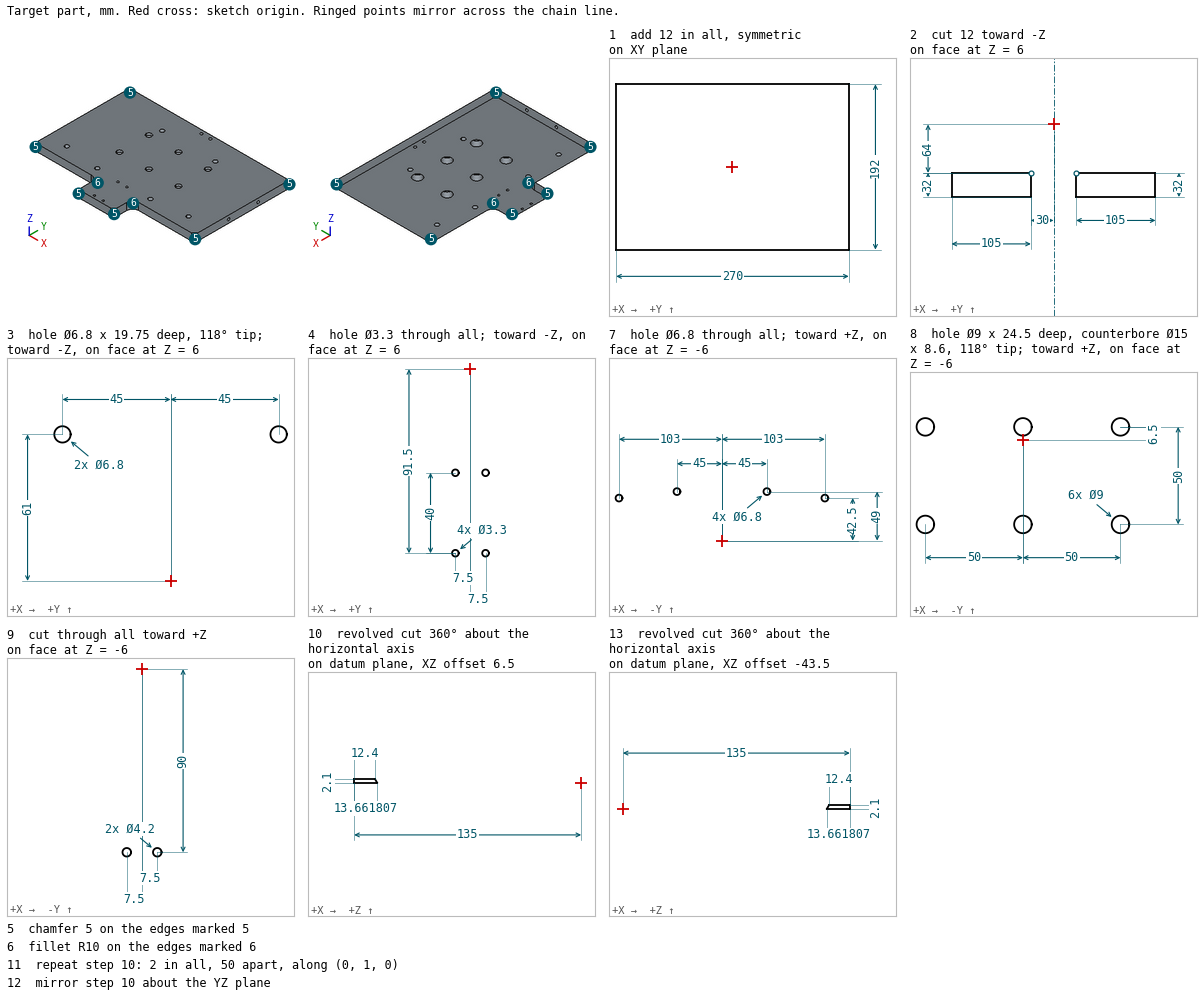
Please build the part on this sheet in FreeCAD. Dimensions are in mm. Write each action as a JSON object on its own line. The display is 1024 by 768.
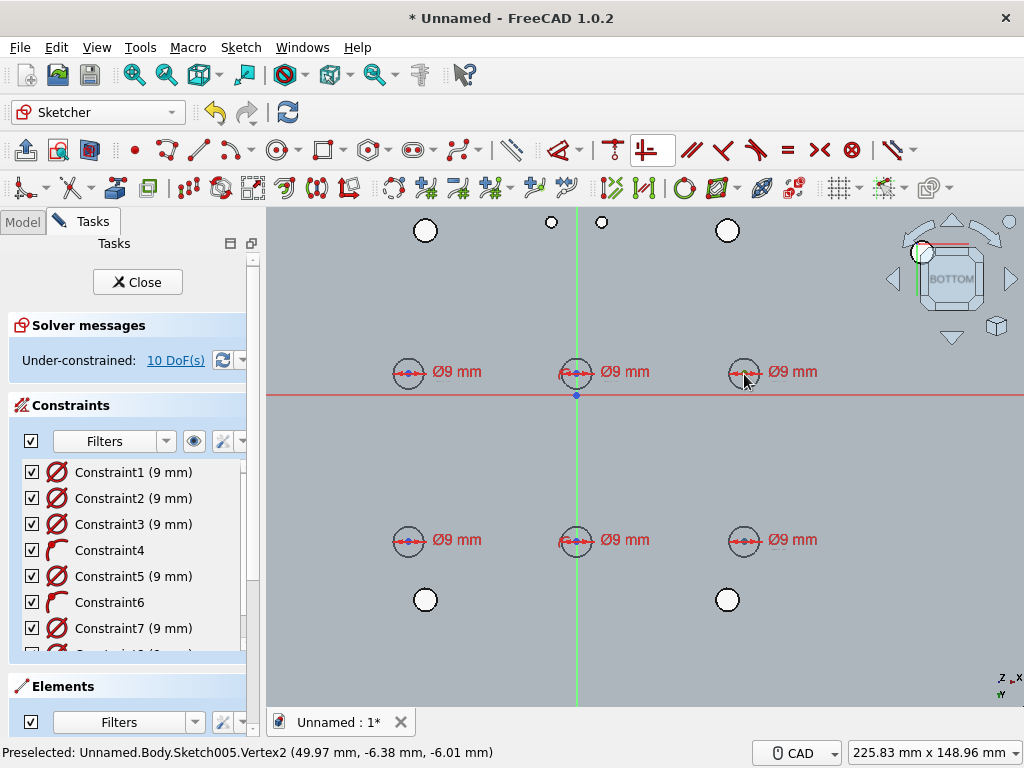
{"action": "key", "text": "v"}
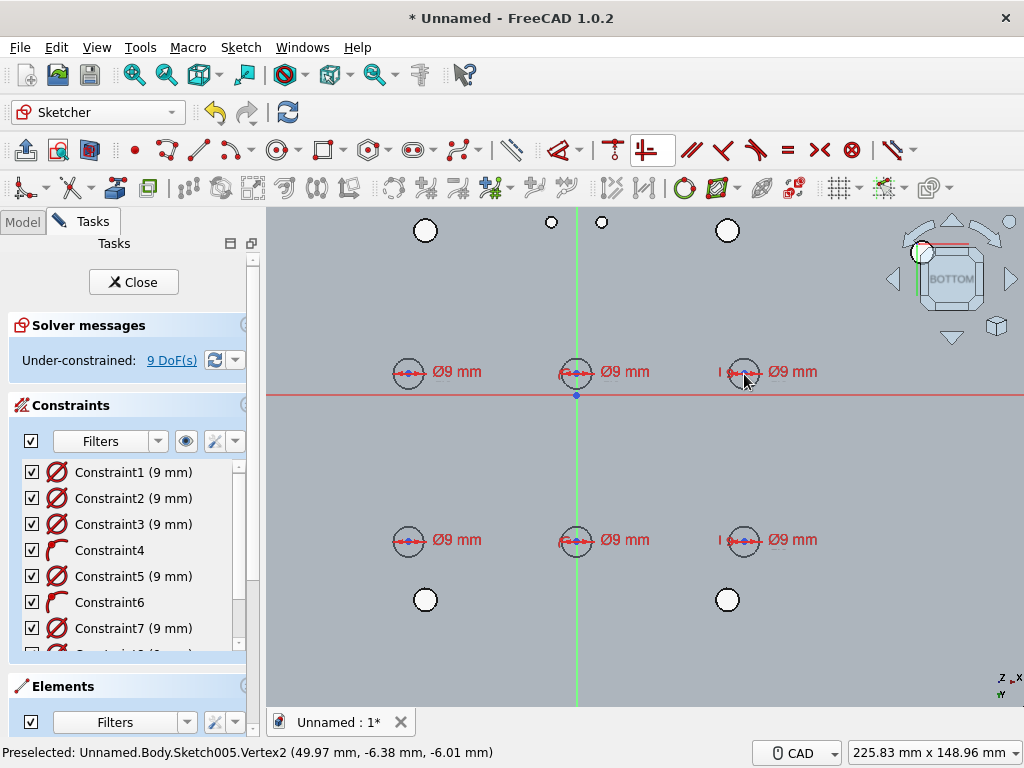
{"action": "left_click", "coordinate": [744, 542]}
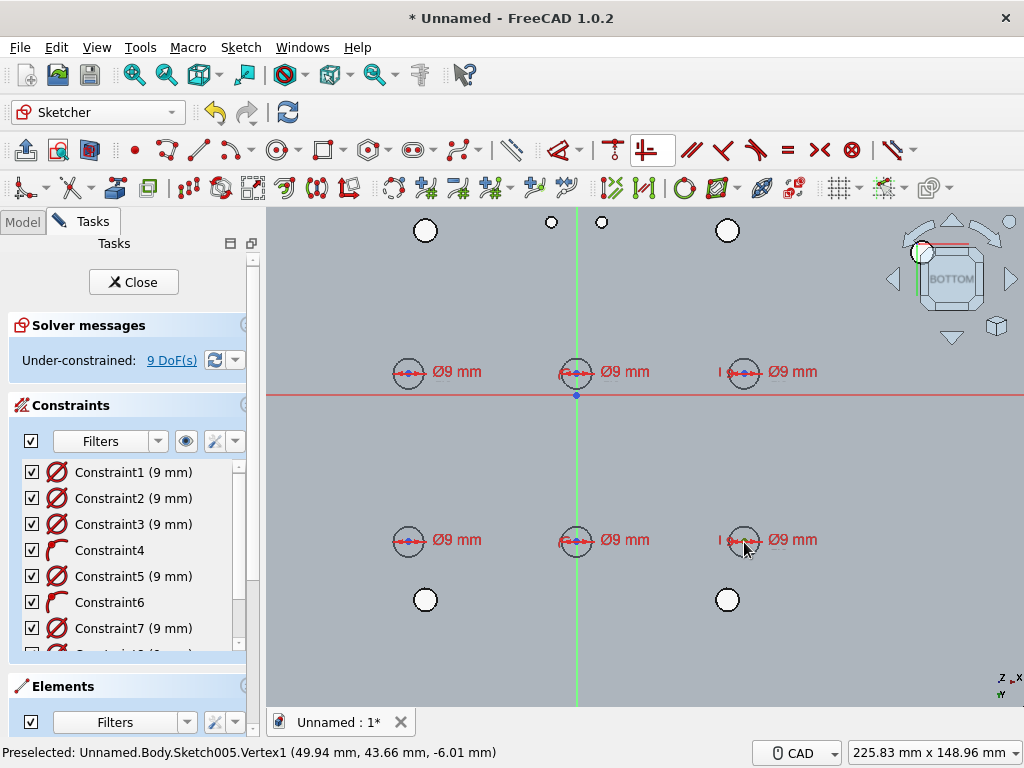
{"action": "left_click", "coordinate": [577, 542]}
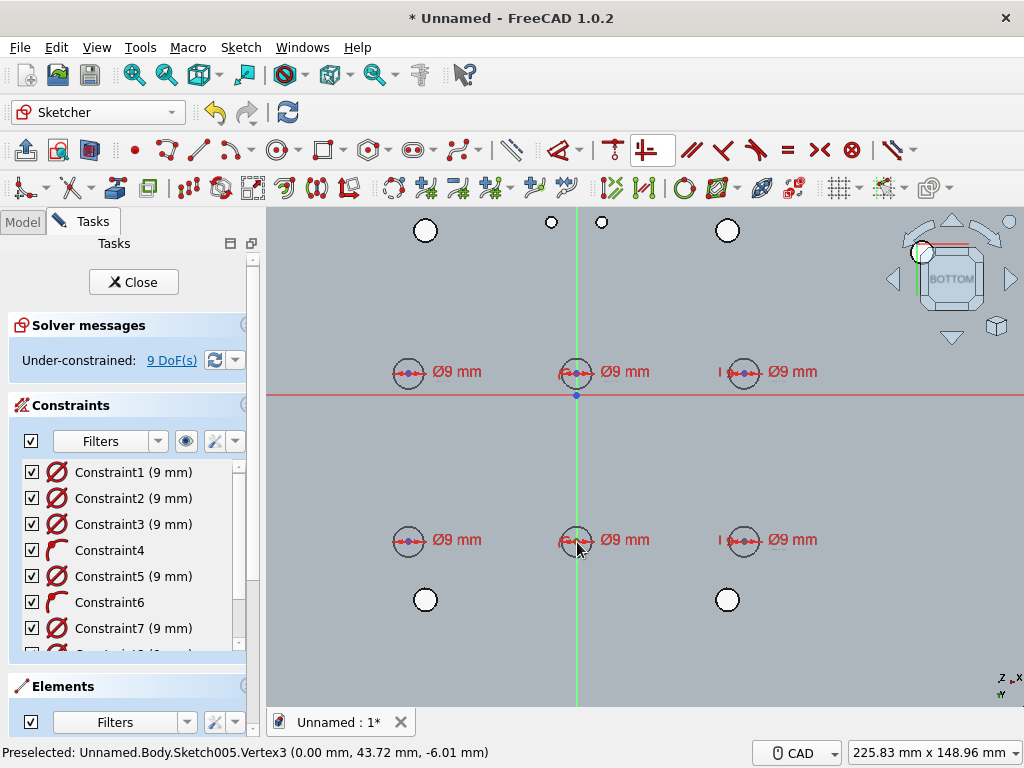
{"action": "key", "text": "h"}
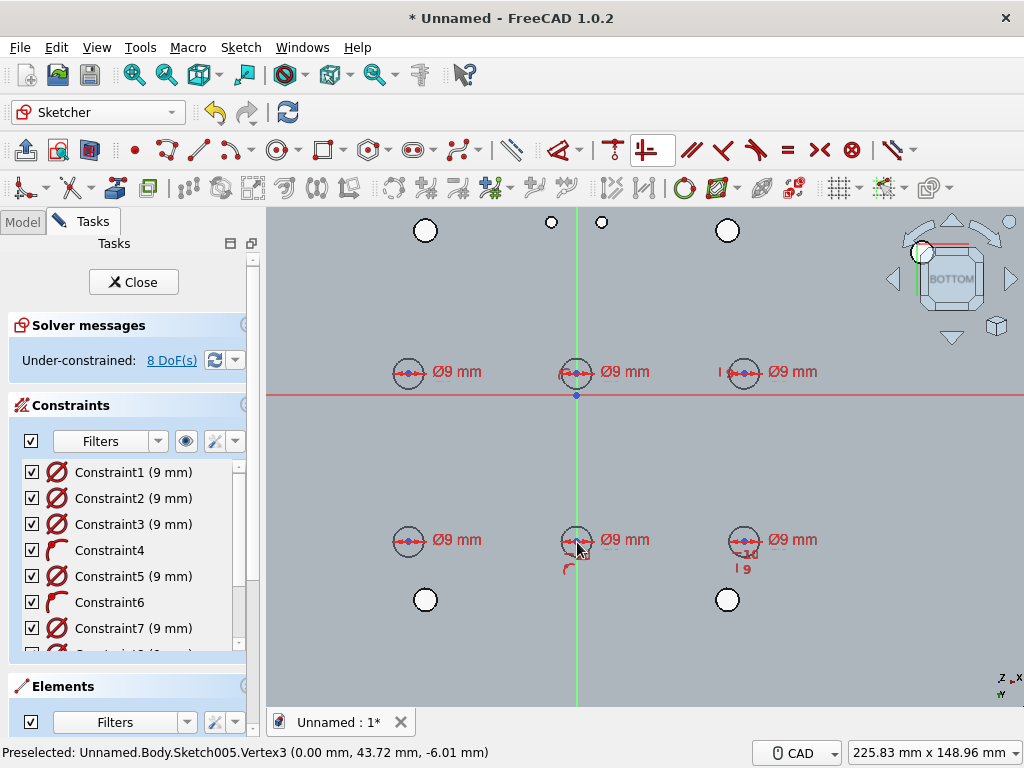
{"action": "left_click", "coordinate": [744, 374]}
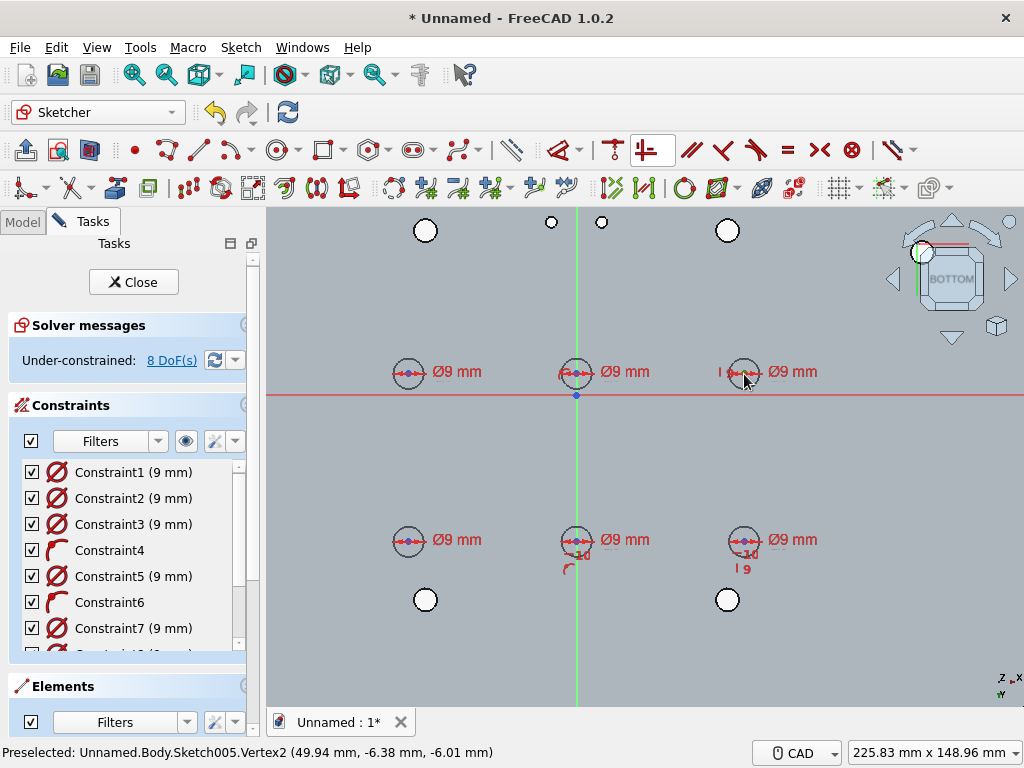
{"action": "left_click", "coordinate": [577, 374]}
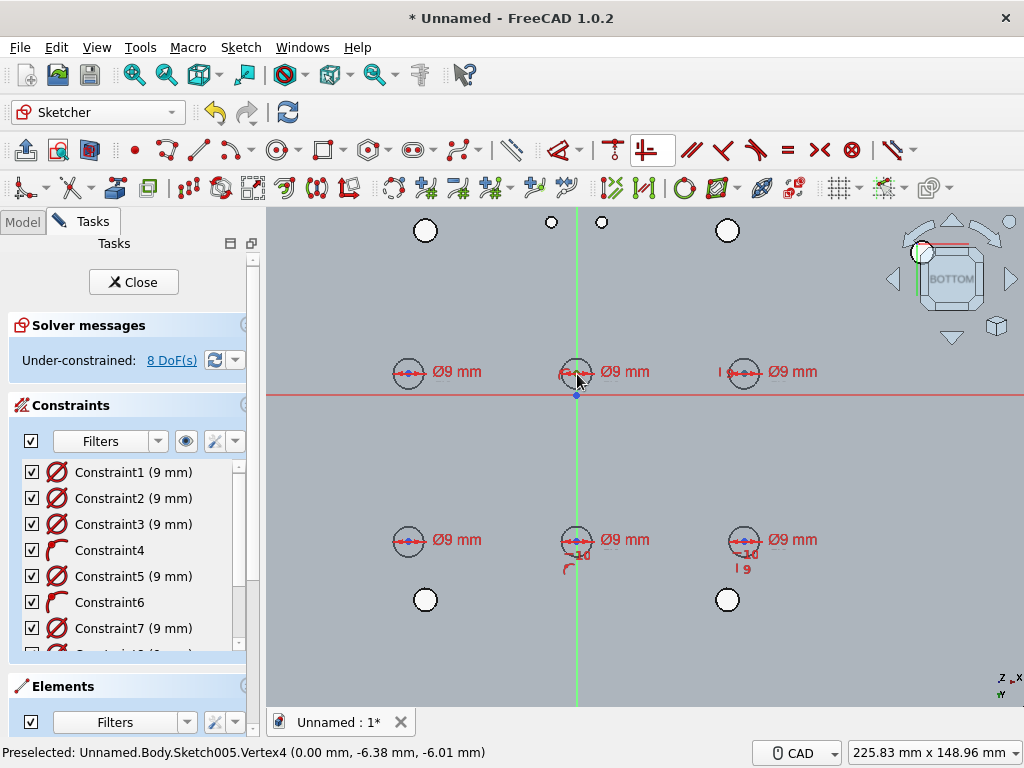
{"action": "key", "text": "h"}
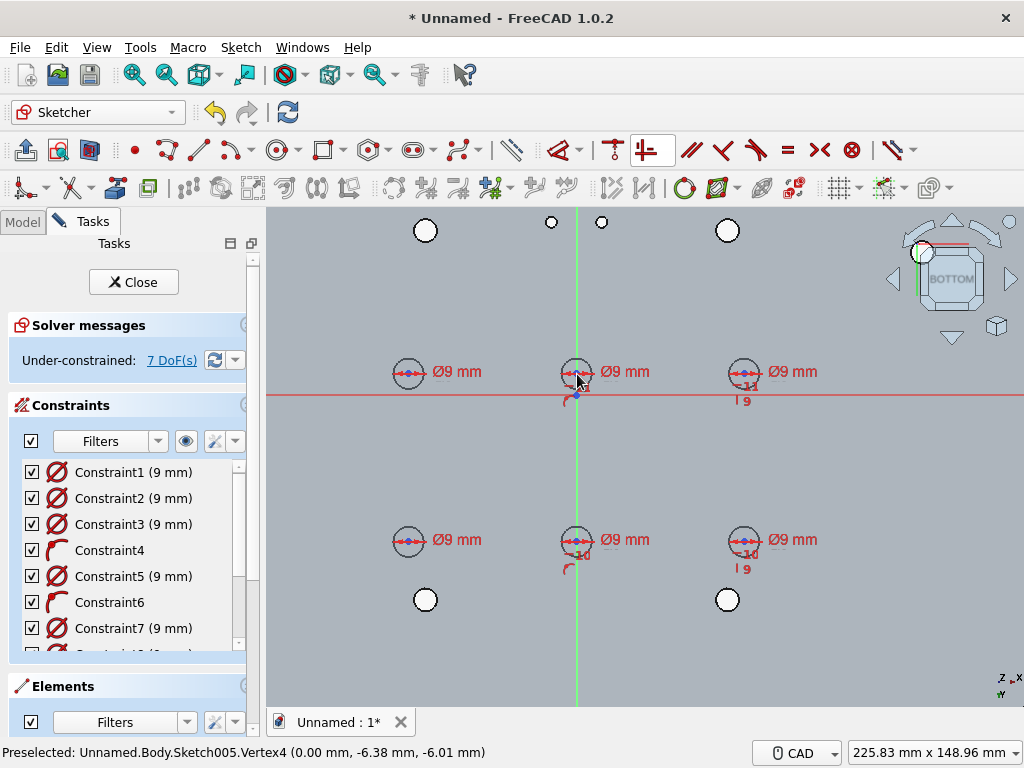
{"action": "left_click", "coordinate": [577, 542]}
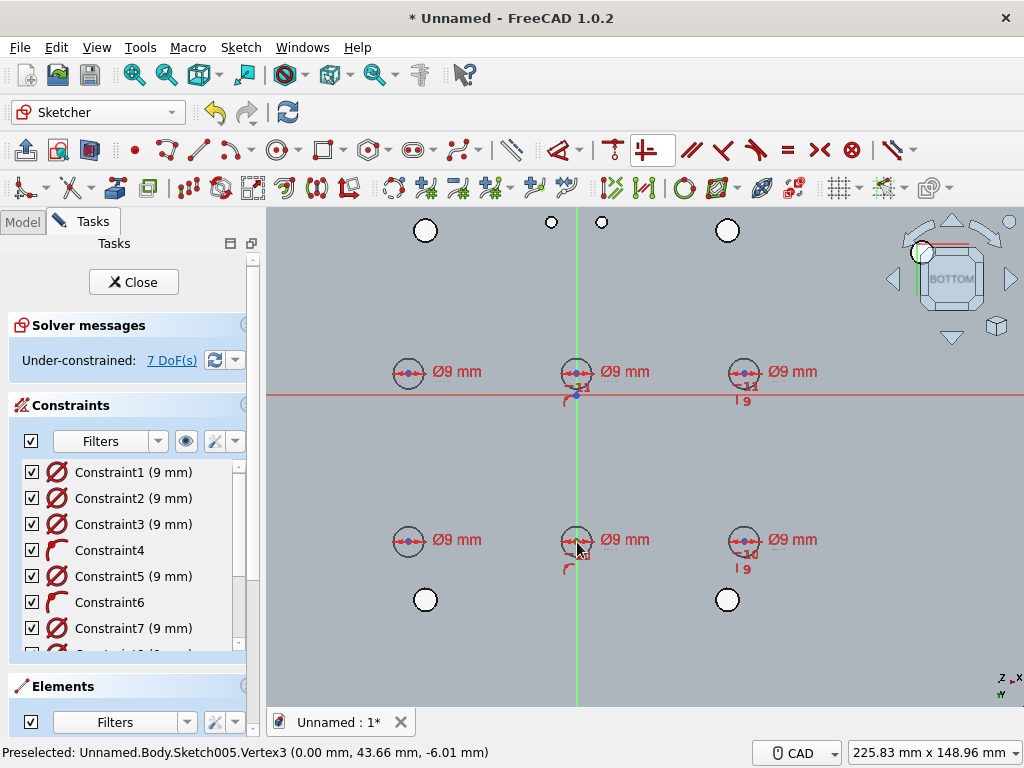
{"action": "left_click", "coordinate": [409, 542]}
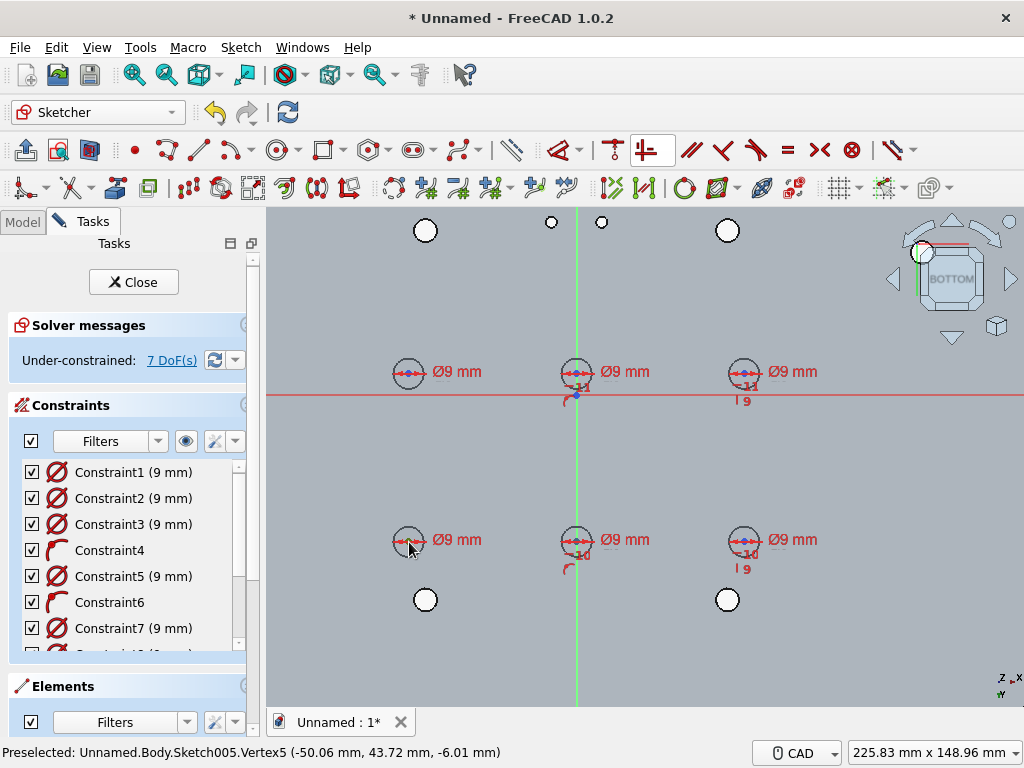
{"action": "key", "text": "h"}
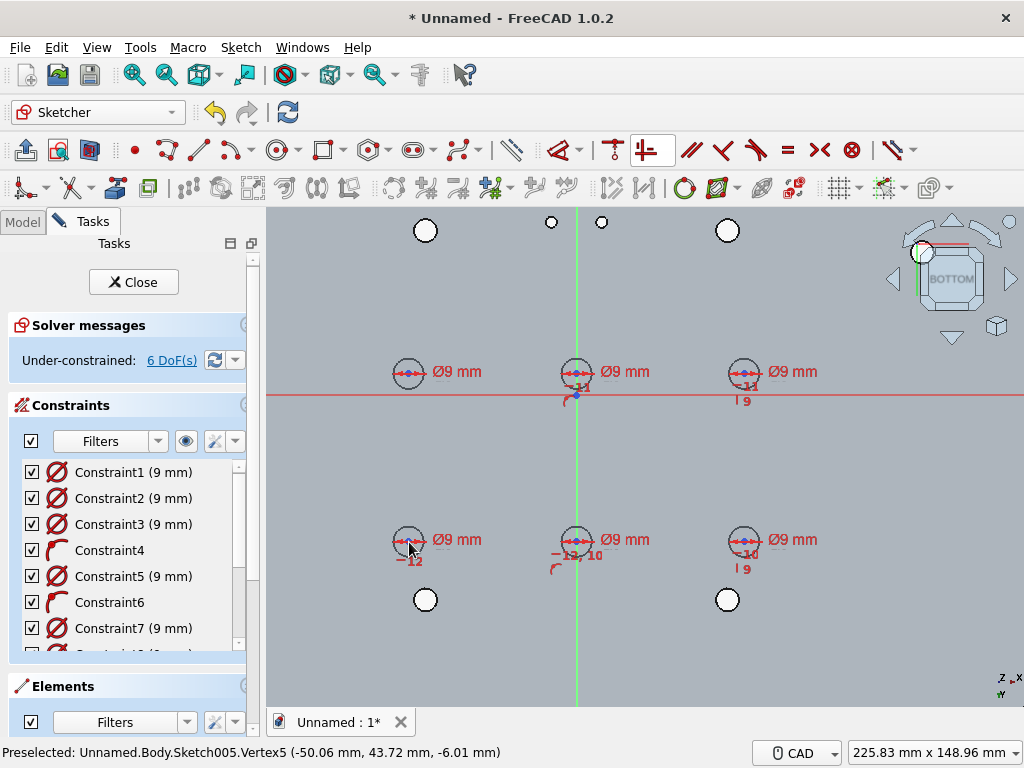
{"action": "left_click", "coordinate": [409, 542]}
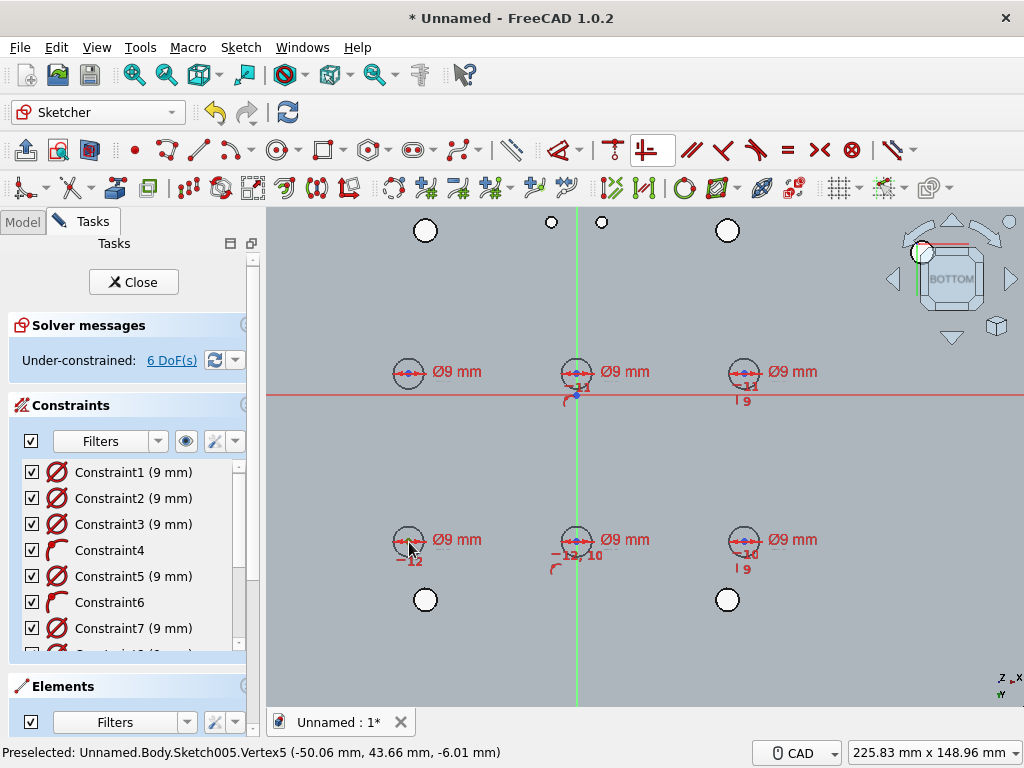
{"action": "left_click", "coordinate": [409, 374]}